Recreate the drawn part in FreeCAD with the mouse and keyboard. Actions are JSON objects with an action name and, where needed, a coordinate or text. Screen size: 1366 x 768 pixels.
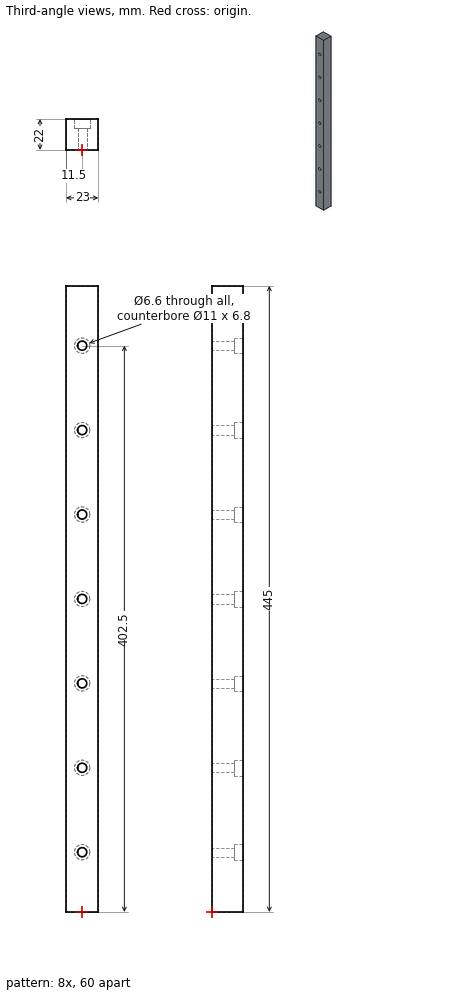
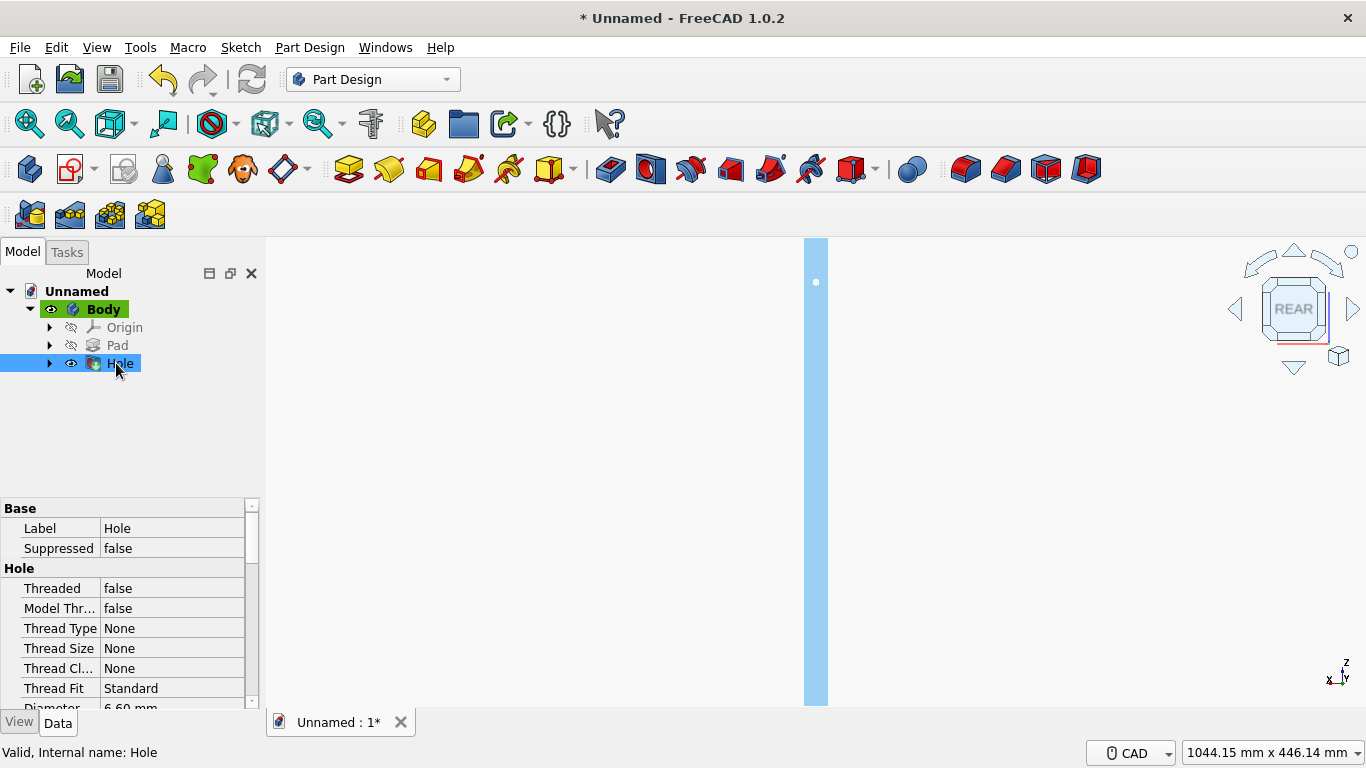
{"action": "left_click", "coordinate": [70, 214]}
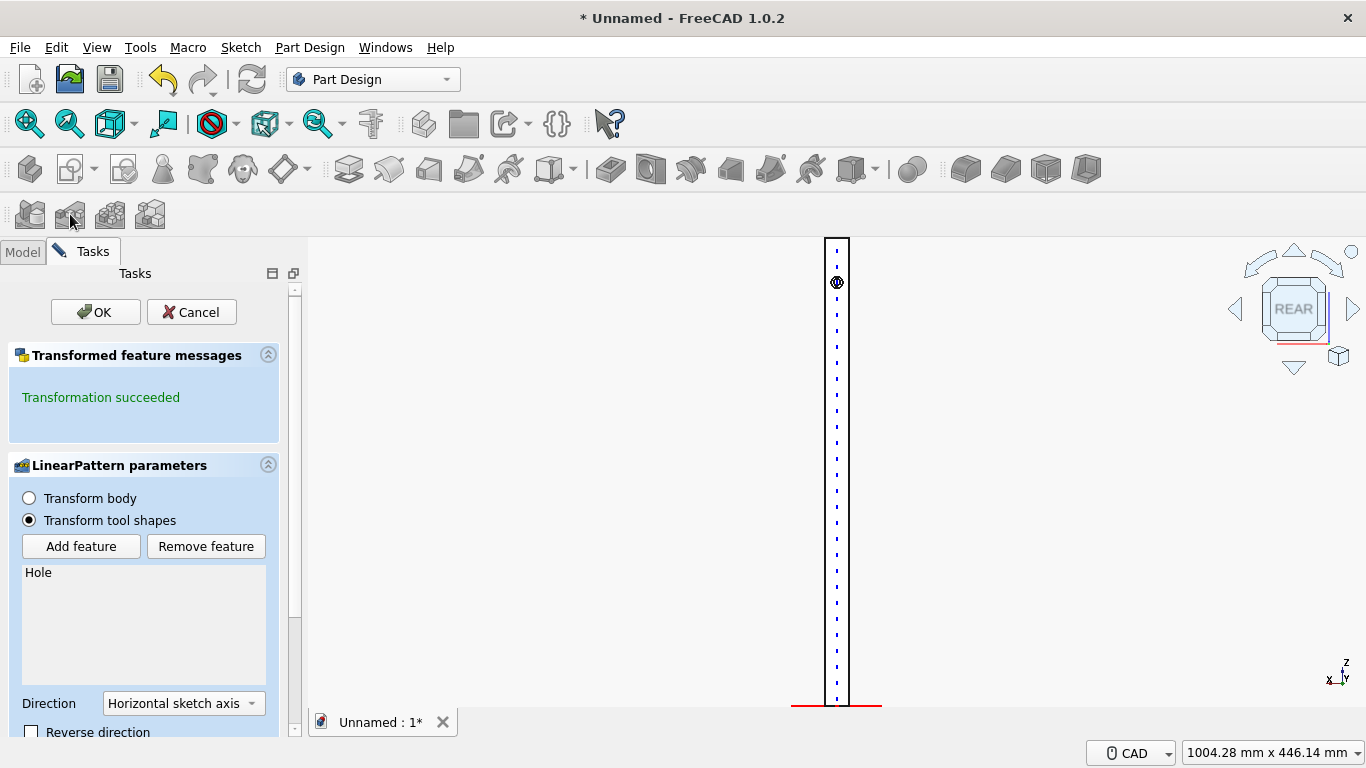
{"action": "left_click", "coordinate": [184, 704]}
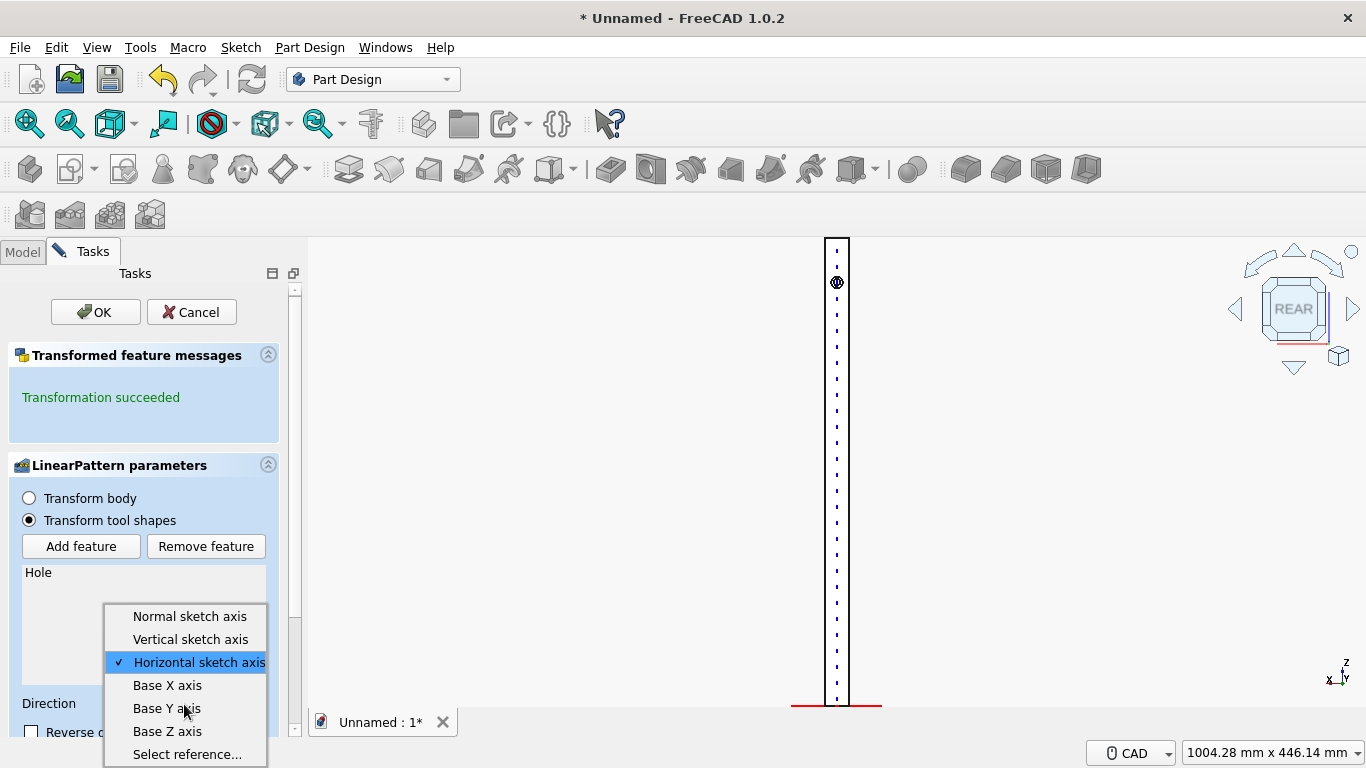
{"action": "left_click", "coordinate": [184, 732]}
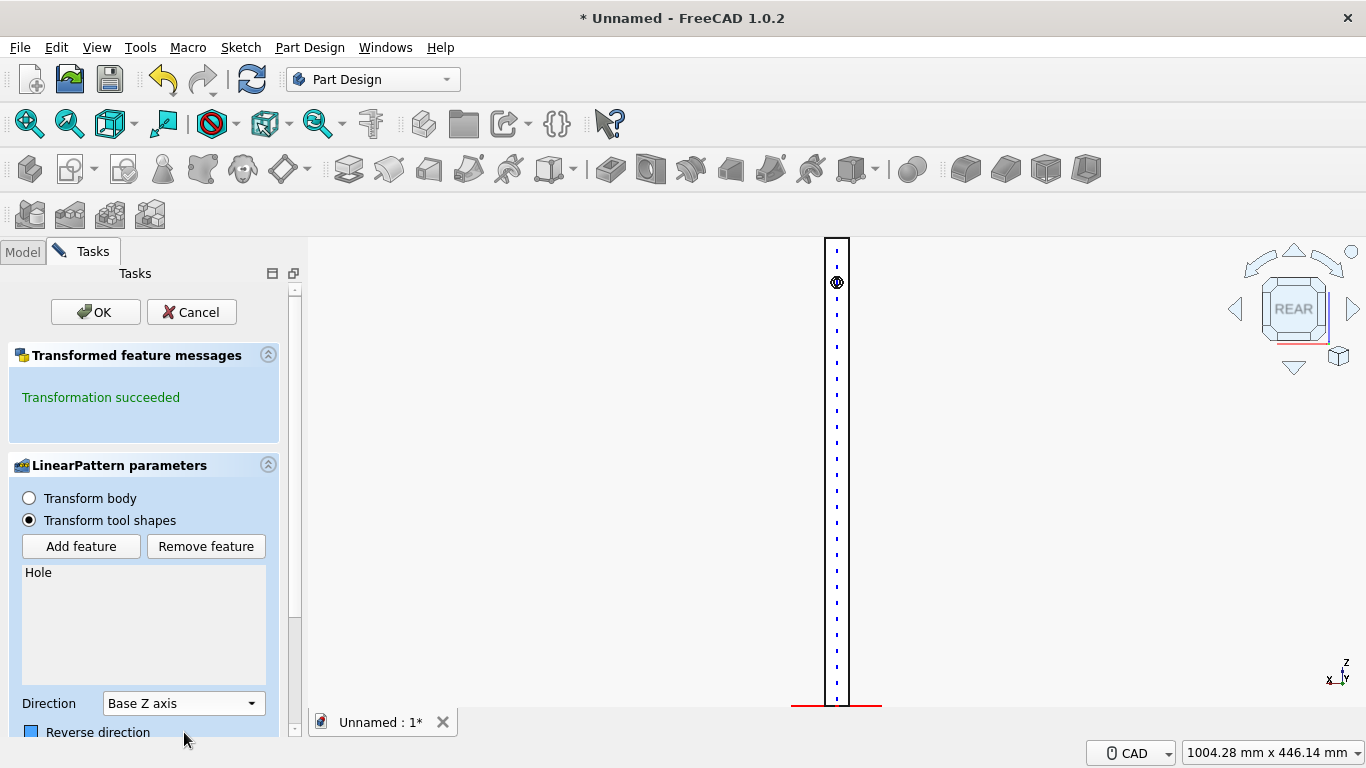
{"action": "scroll", "coordinate": [295, 510], "scroll_direction": "down", "scroll_amount": 2}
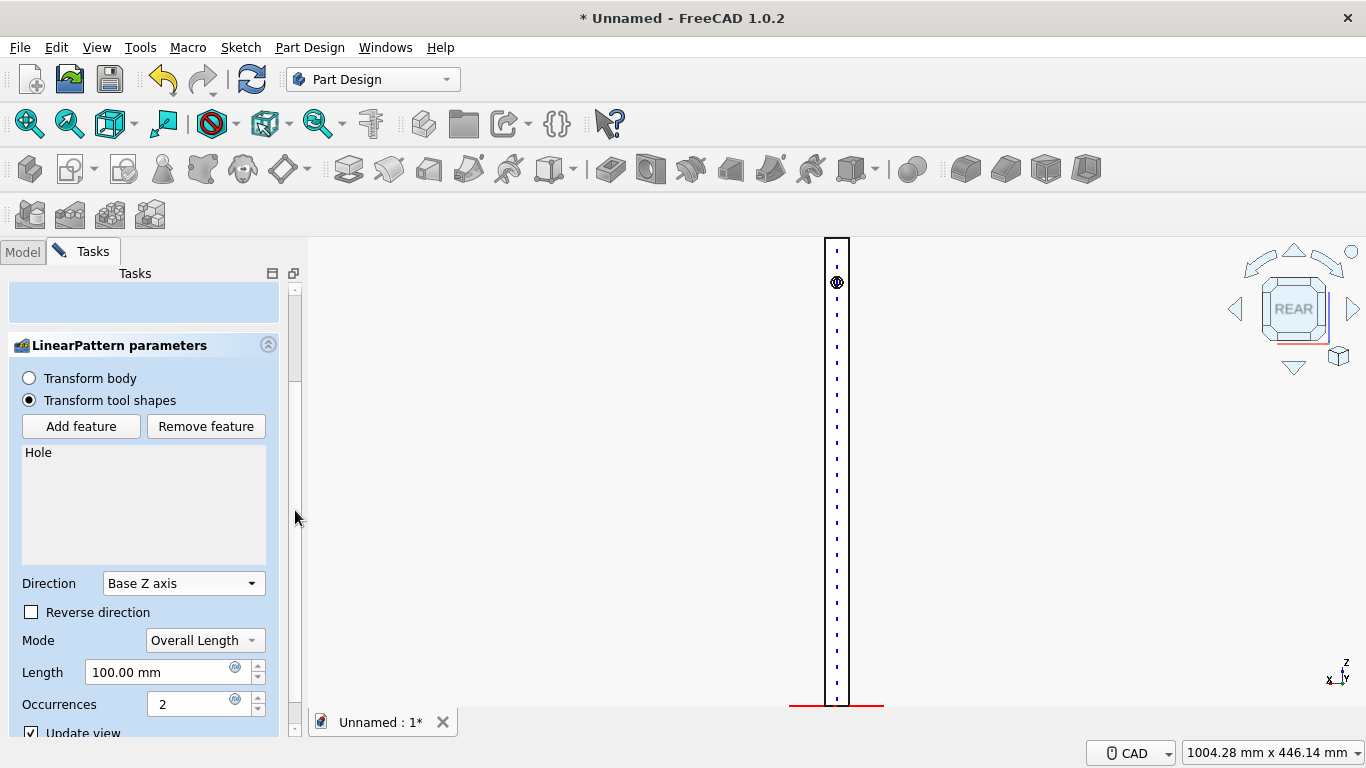
{"action": "left_click", "coordinate": [206, 640]}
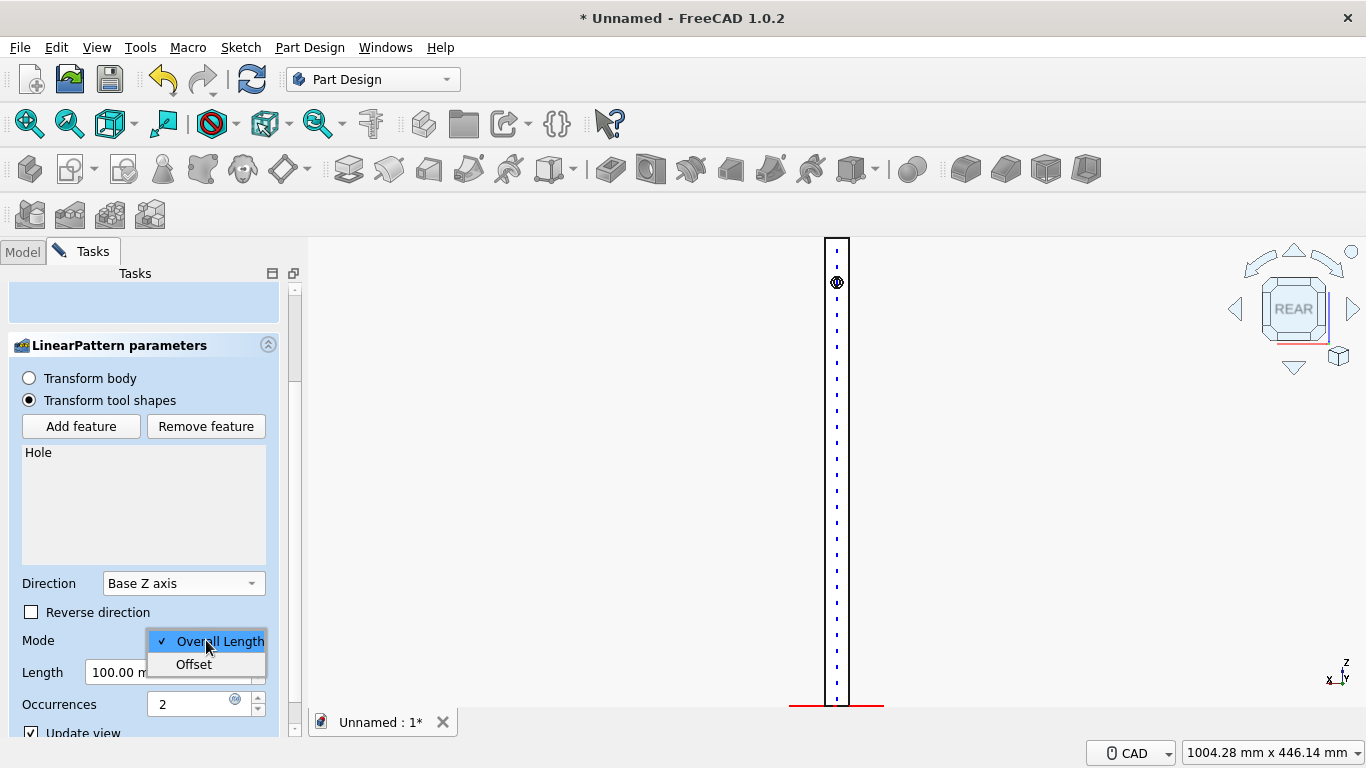
{"action": "left_click", "coordinate": [206, 664]}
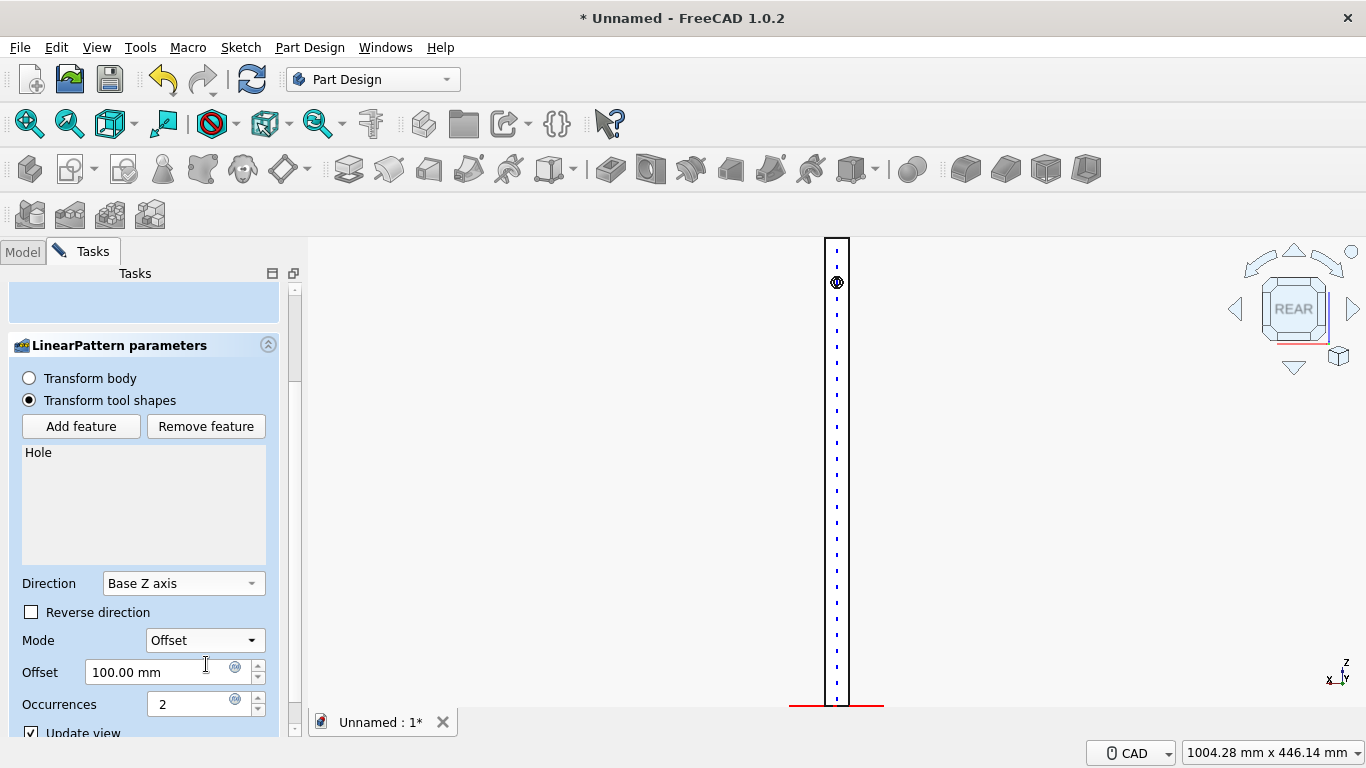
{"action": "triple_click", "coordinate": [168, 672]}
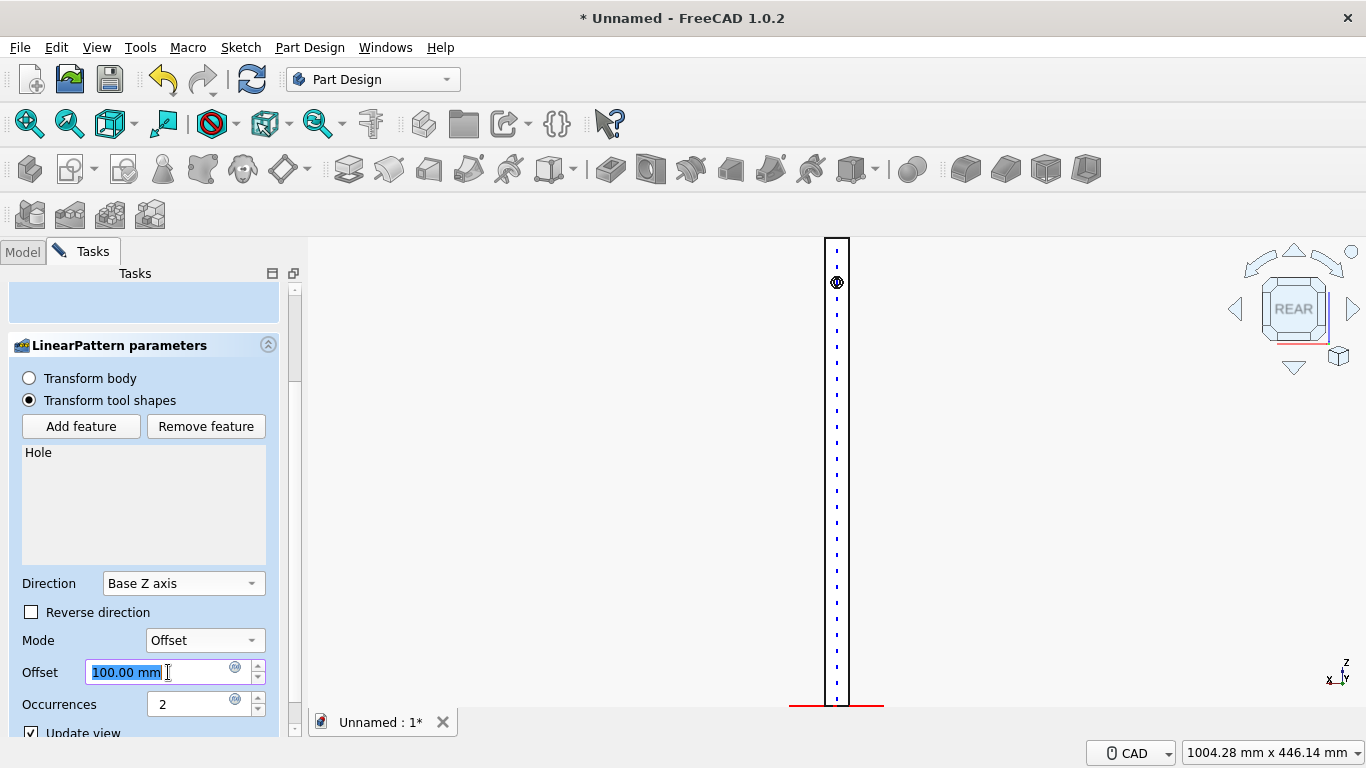
{"action": "type", "text": "60"}
{"action": "key", "text": "Tab"}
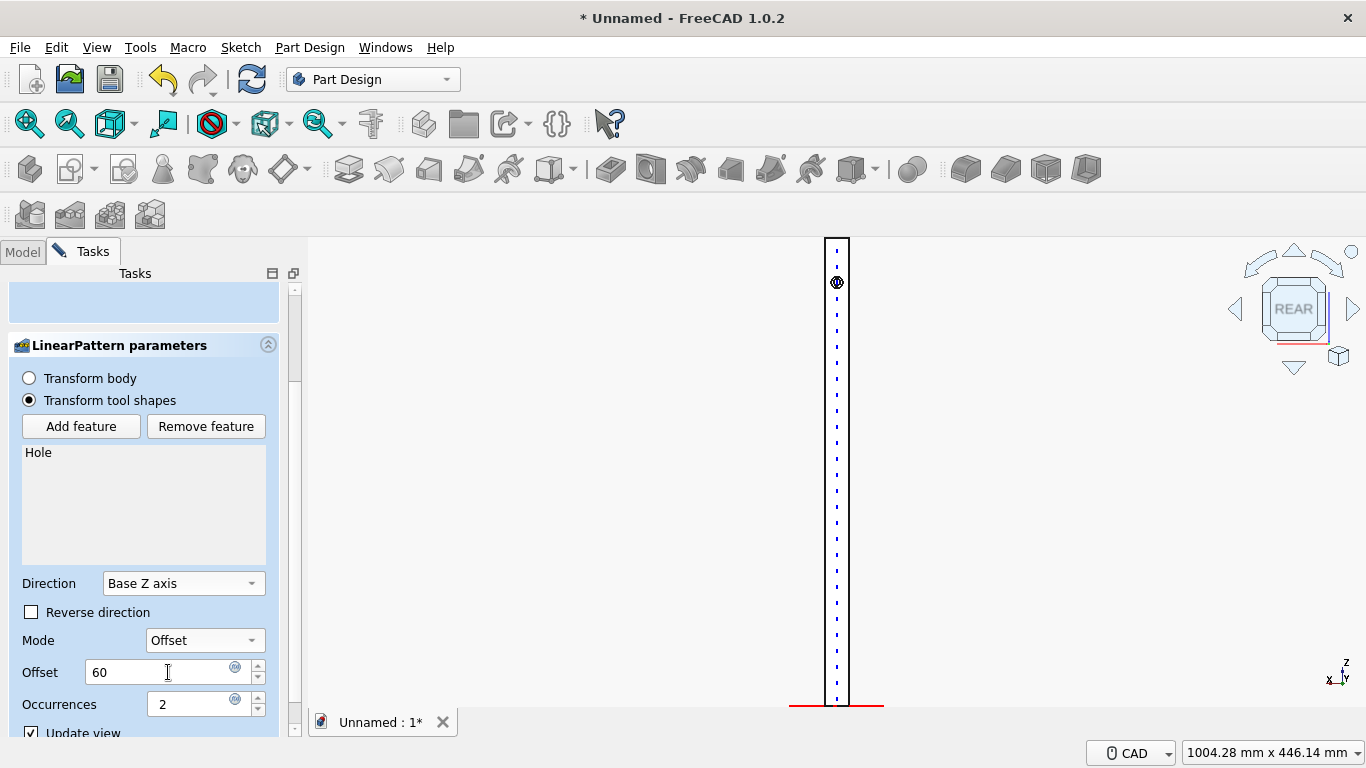
{"action": "triple_click", "coordinate": [198, 704]}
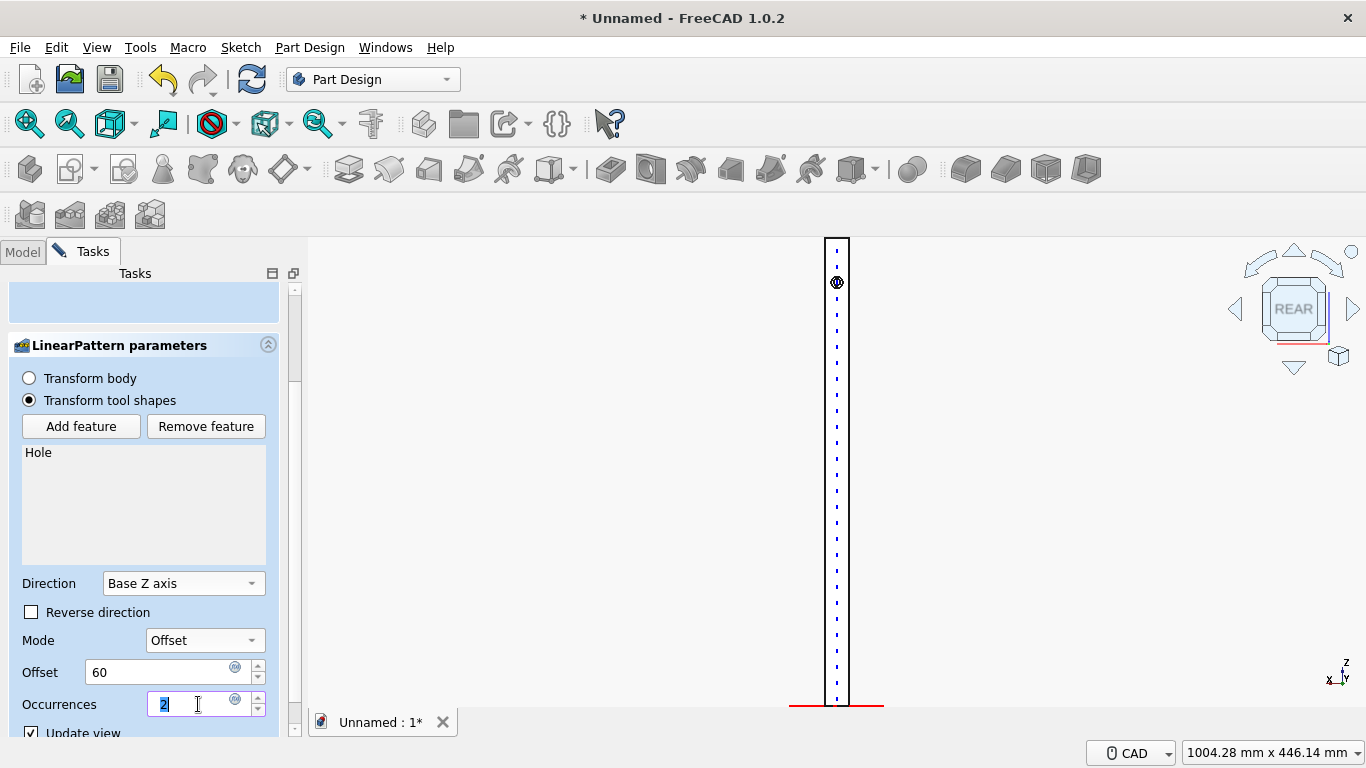
{"action": "type", "text": "8"}
{"action": "key", "text": "Tab"}